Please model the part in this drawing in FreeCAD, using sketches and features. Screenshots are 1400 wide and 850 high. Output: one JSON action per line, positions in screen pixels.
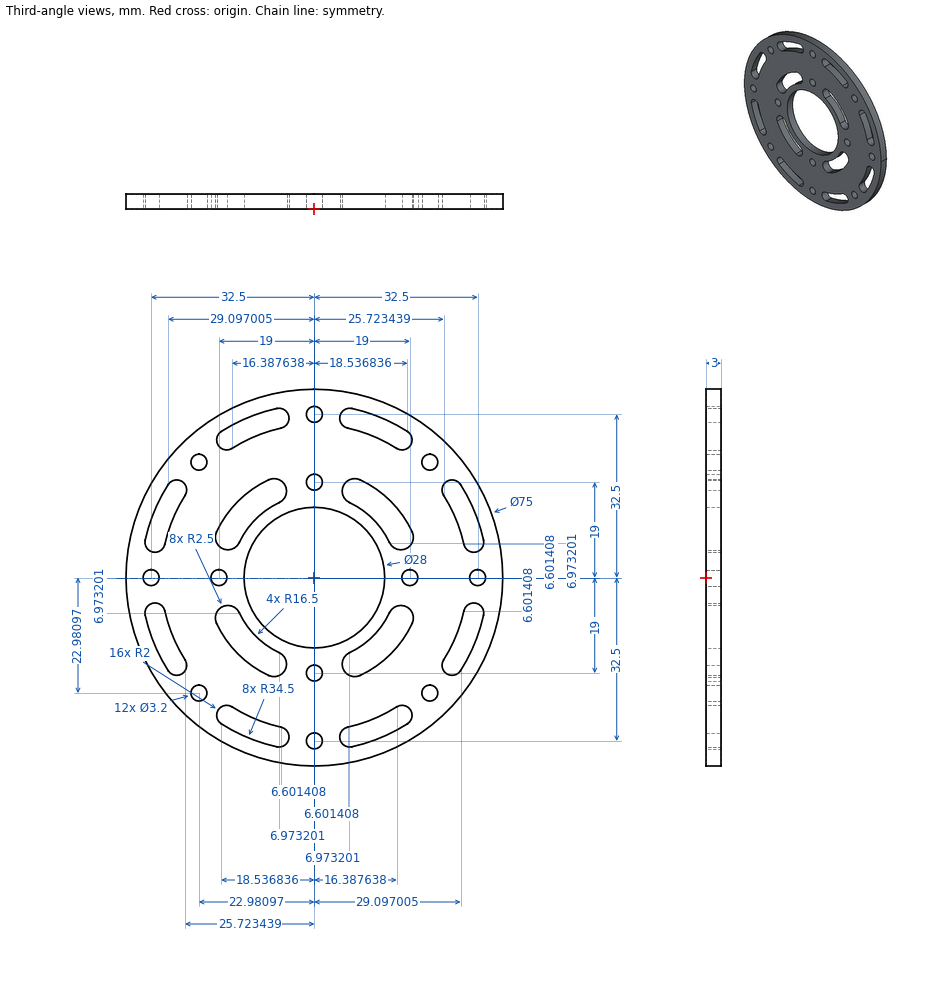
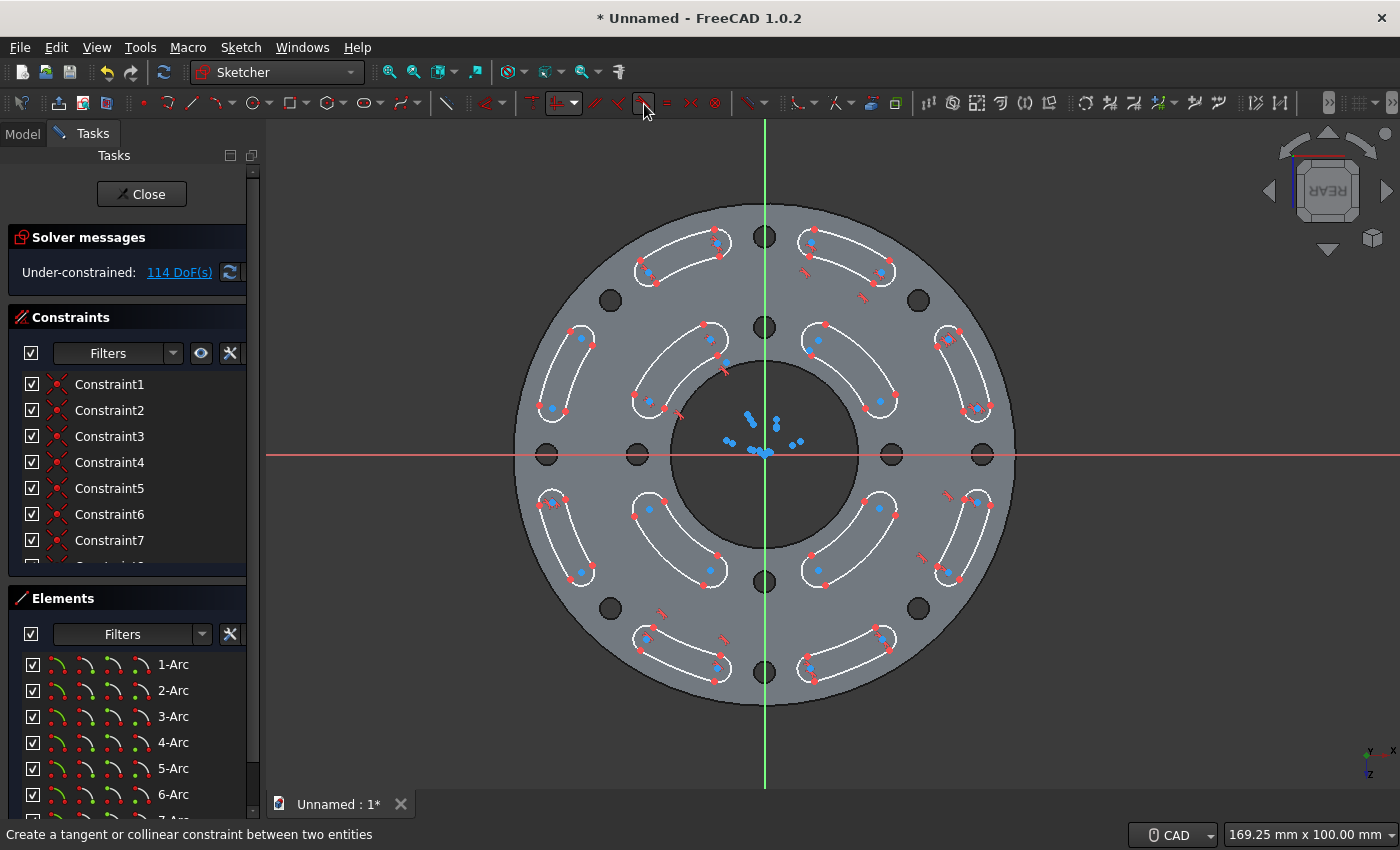
{"action": "left_click", "coordinate": [546, 529]}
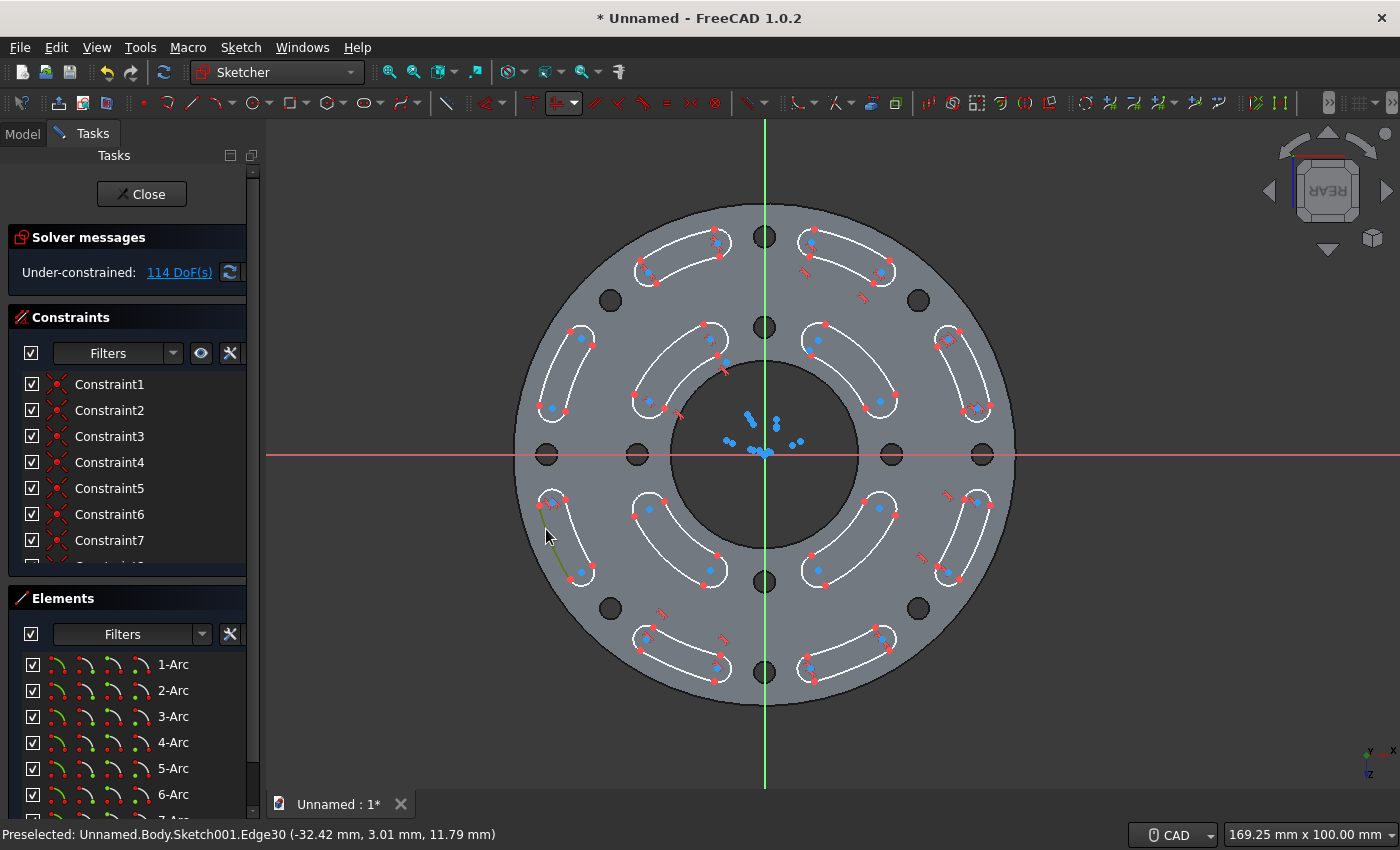
{"action": "left_click", "coordinate": [580, 586]}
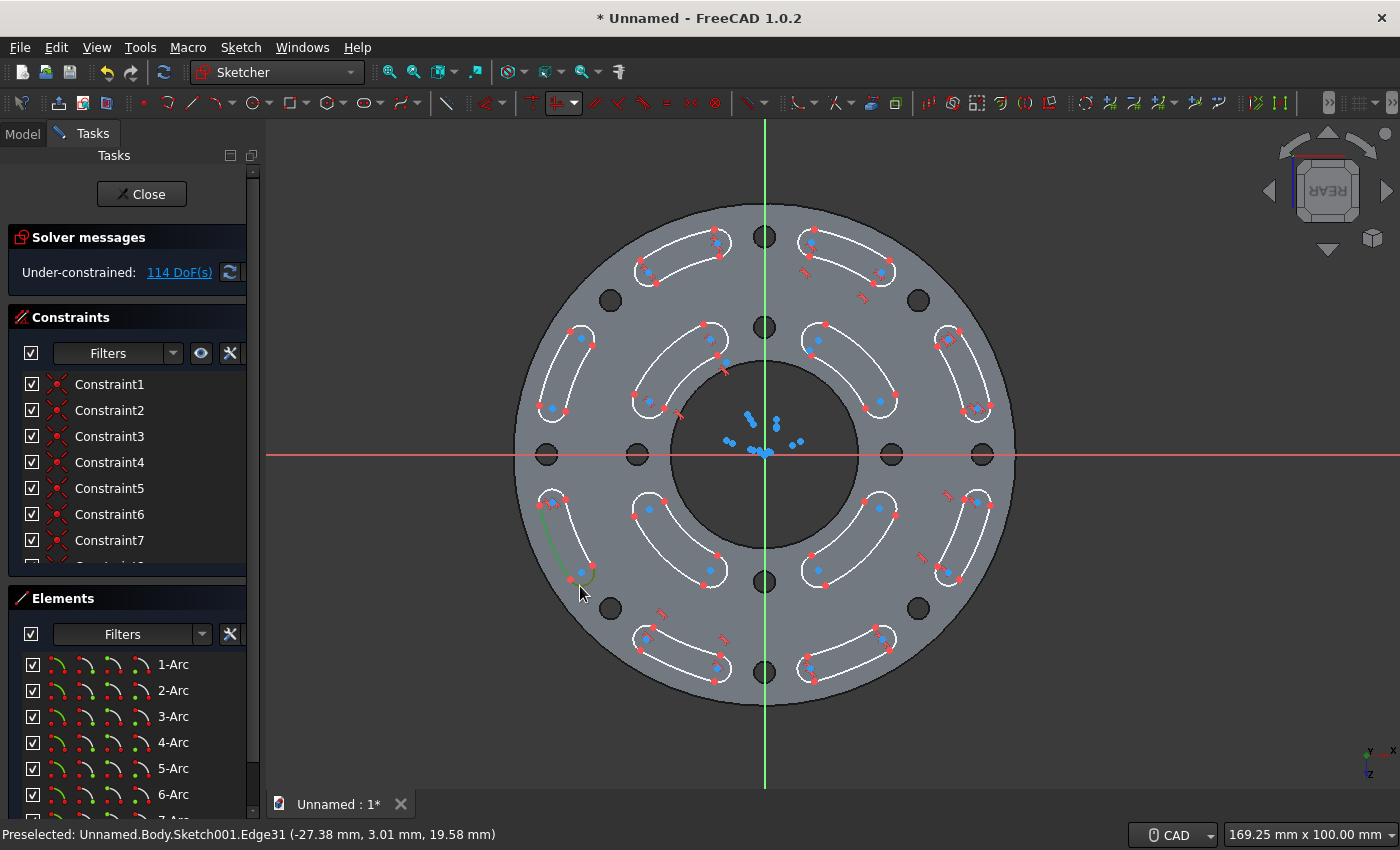
{"action": "left_click", "coordinate": [644, 104]}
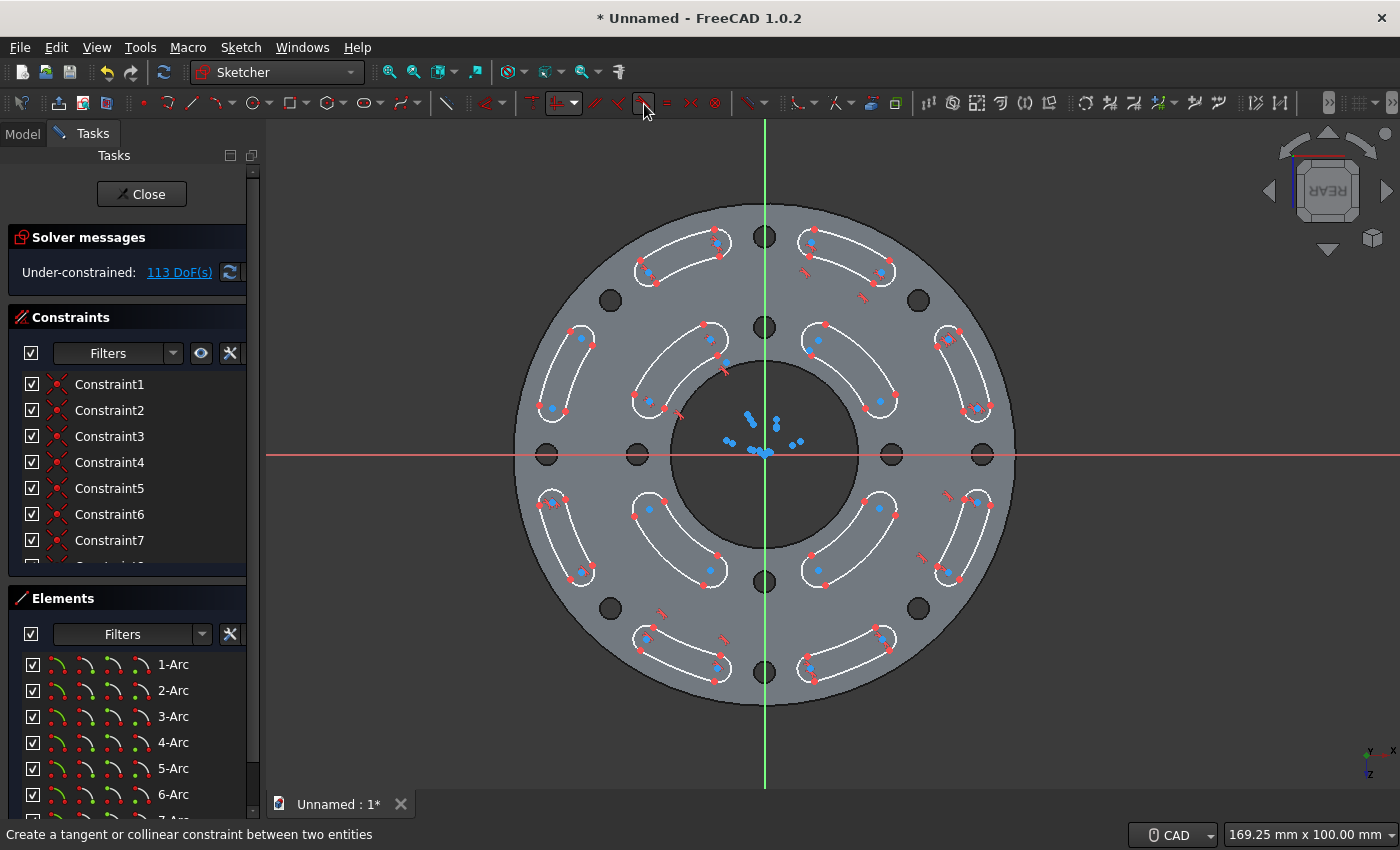
{"action": "left_click", "coordinate": [580, 586]}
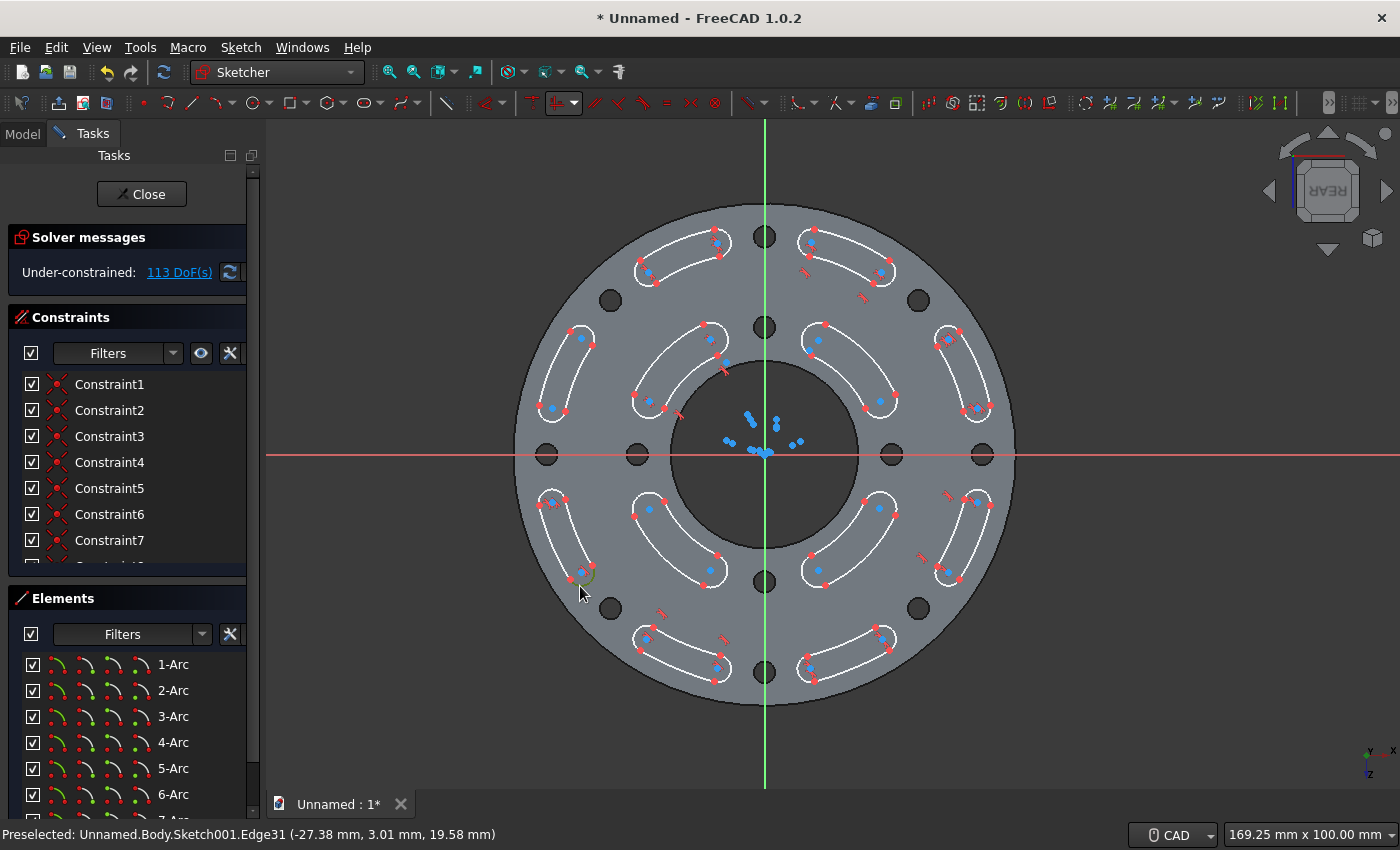
{"action": "left_click", "coordinate": [571, 520]}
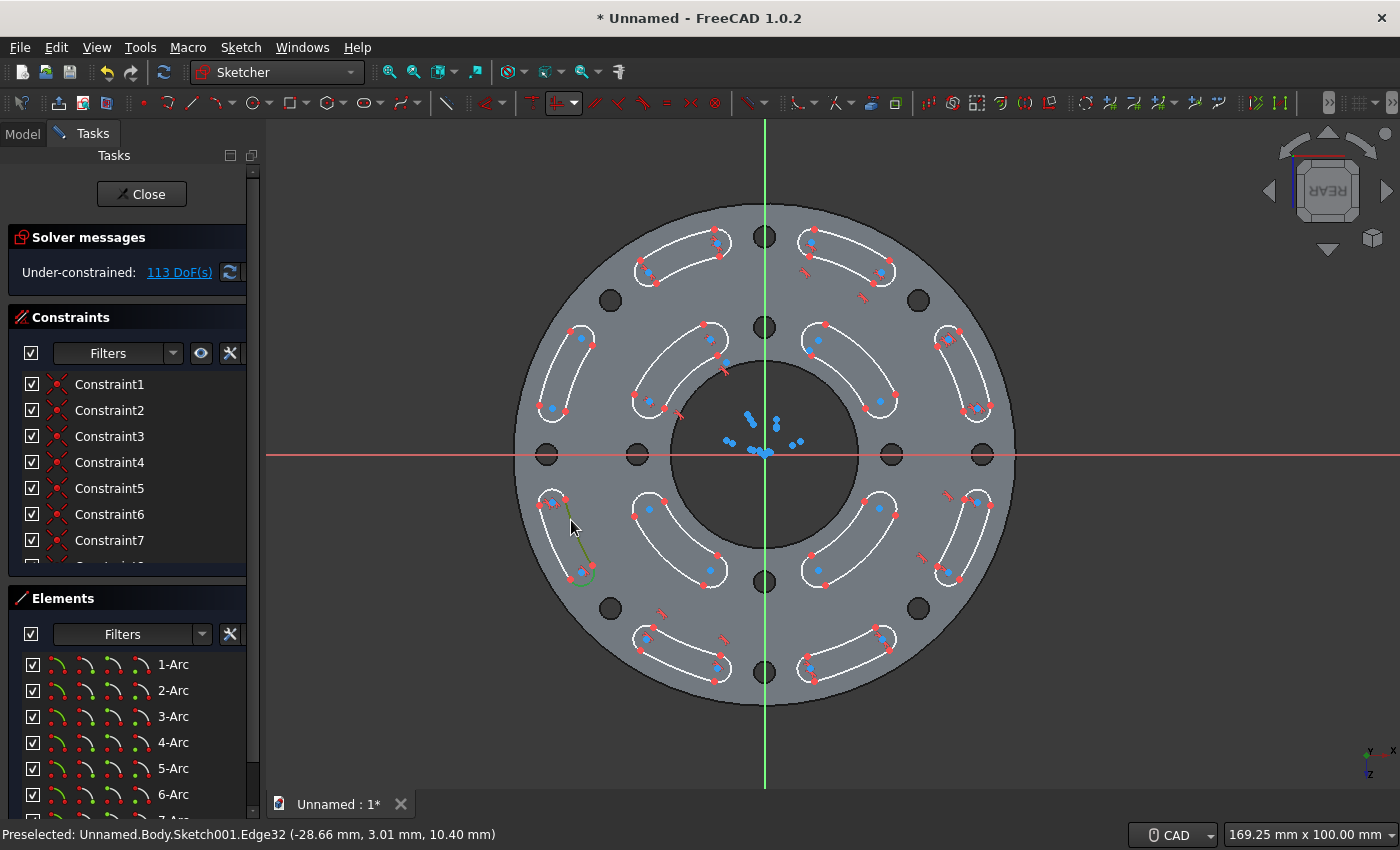
{"action": "left_click", "coordinate": [644, 104]}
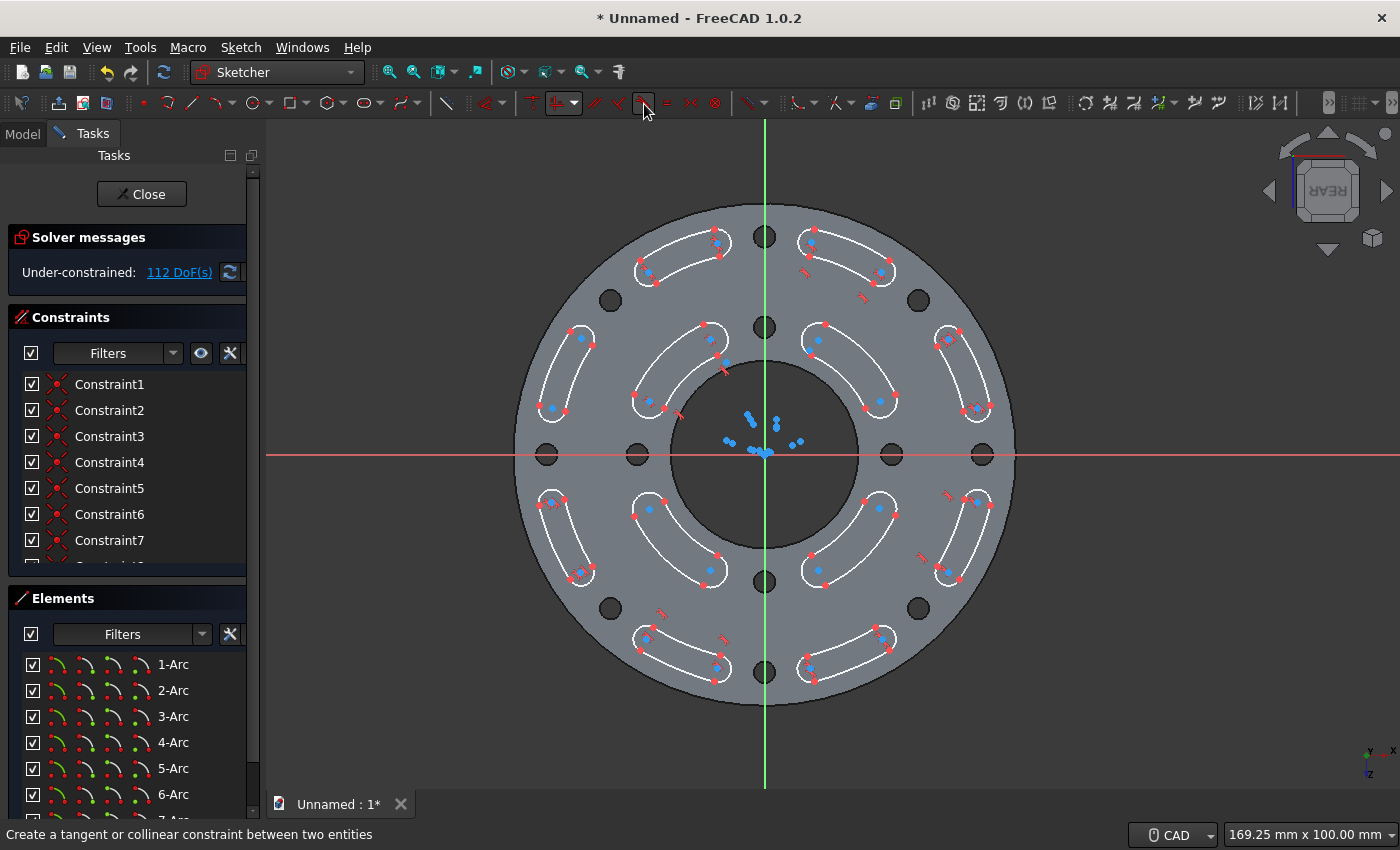
{"action": "left_click", "coordinate": [581, 364]}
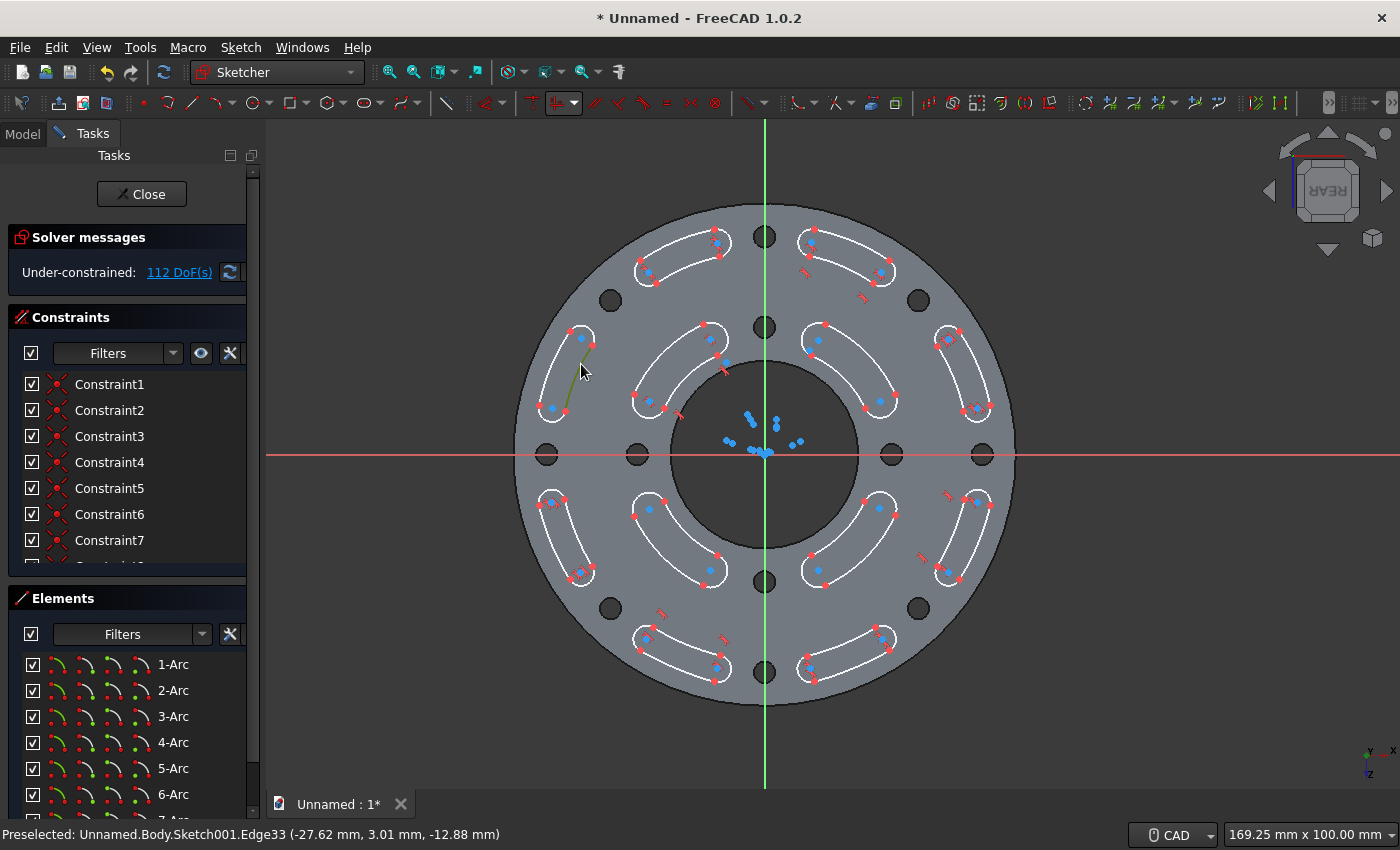
{"action": "left_click", "coordinate": [593, 334]}